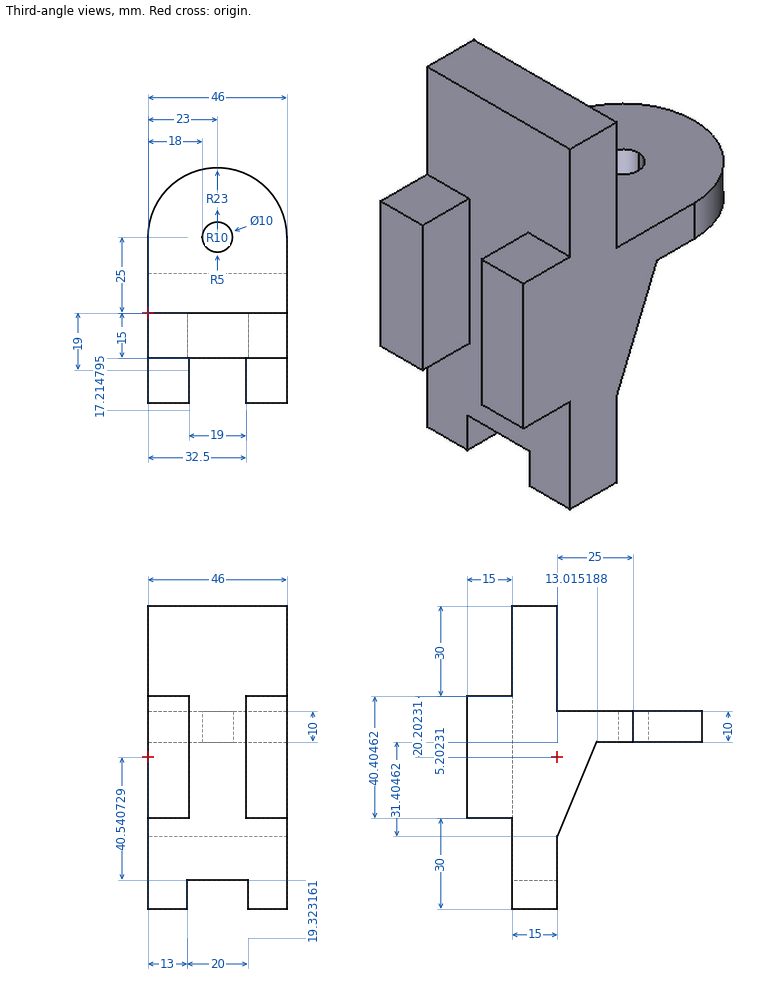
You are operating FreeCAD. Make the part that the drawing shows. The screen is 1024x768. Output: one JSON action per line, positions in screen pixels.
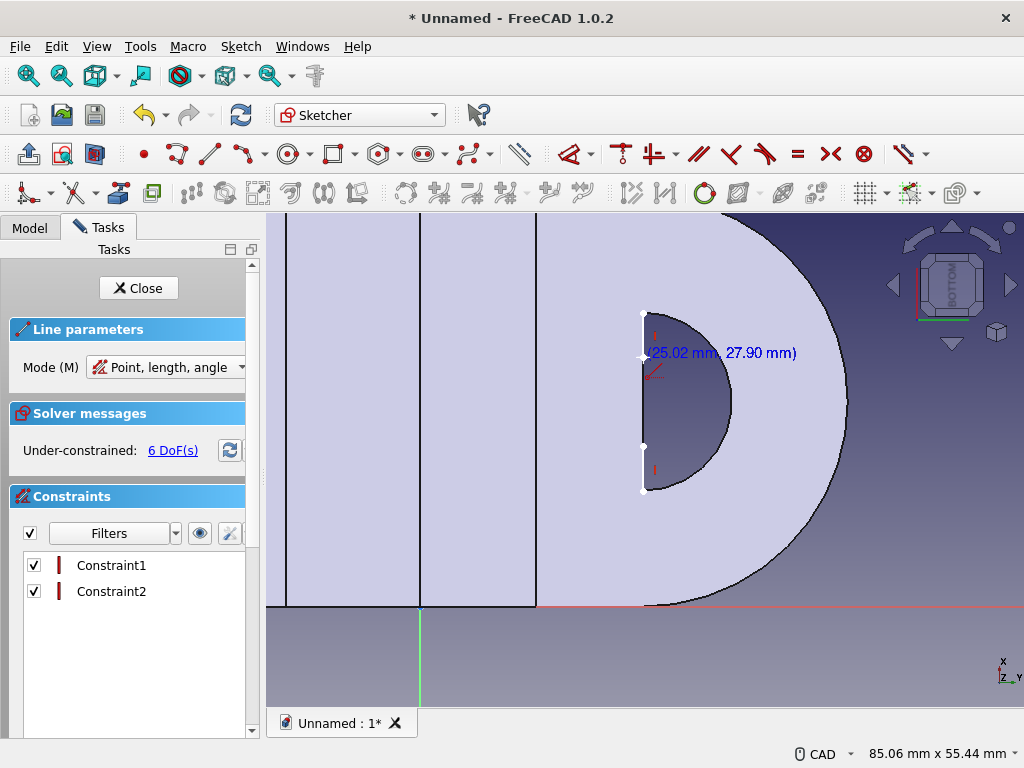
{"action": "key", "text": "g 3 a"}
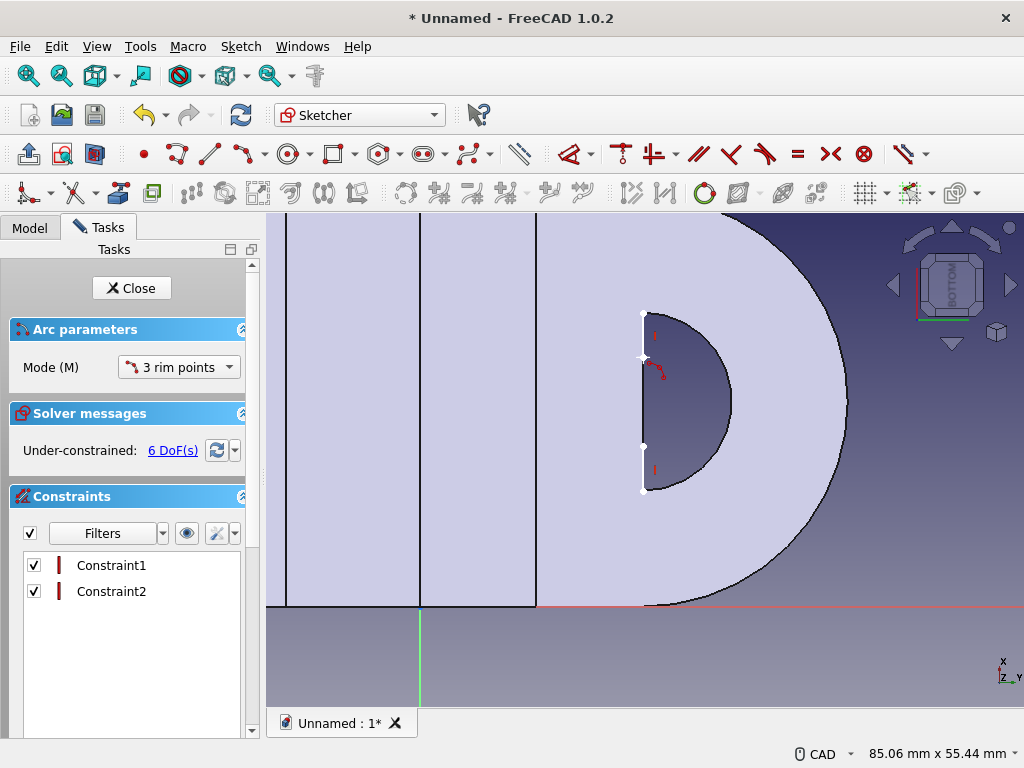
{"action": "left_click", "coordinate": [643, 492]}
{"action": "left_click", "coordinate": [643, 314]}
{"action": "left_click", "coordinate": [732, 402]}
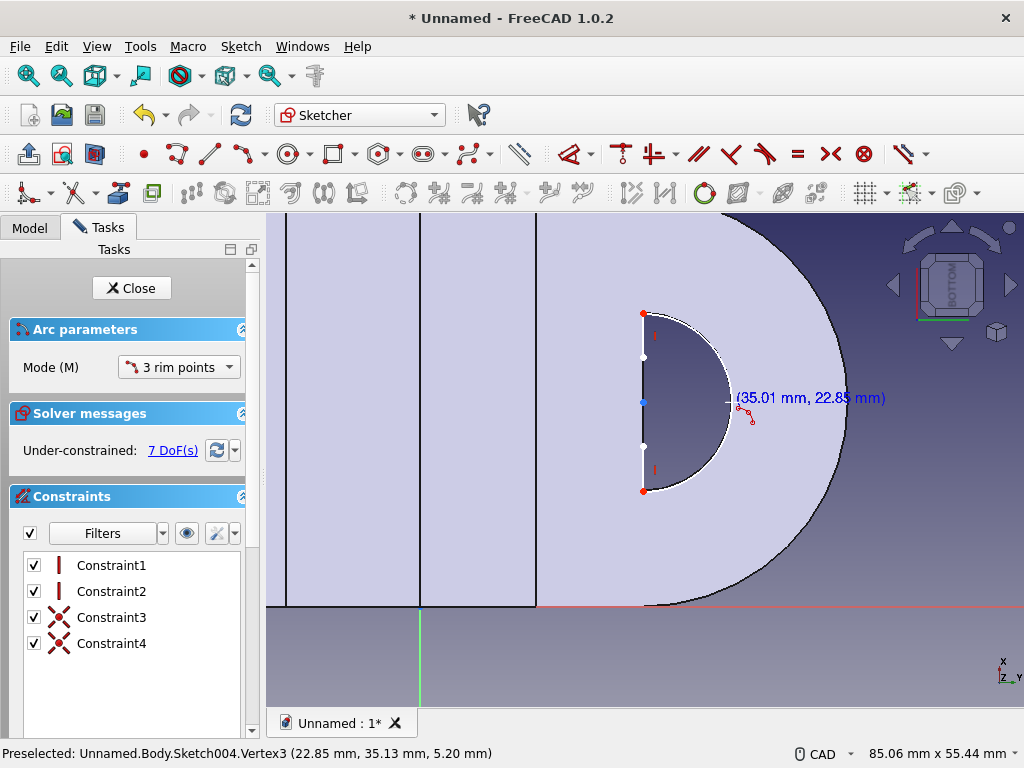
{"action": "left_click", "coordinate": [643, 358]}
{"action": "left_click", "coordinate": [643, 447]}
{"action": "left_click", "coordinate": [598, 402]}
{"action": "key", "text": "Escape"}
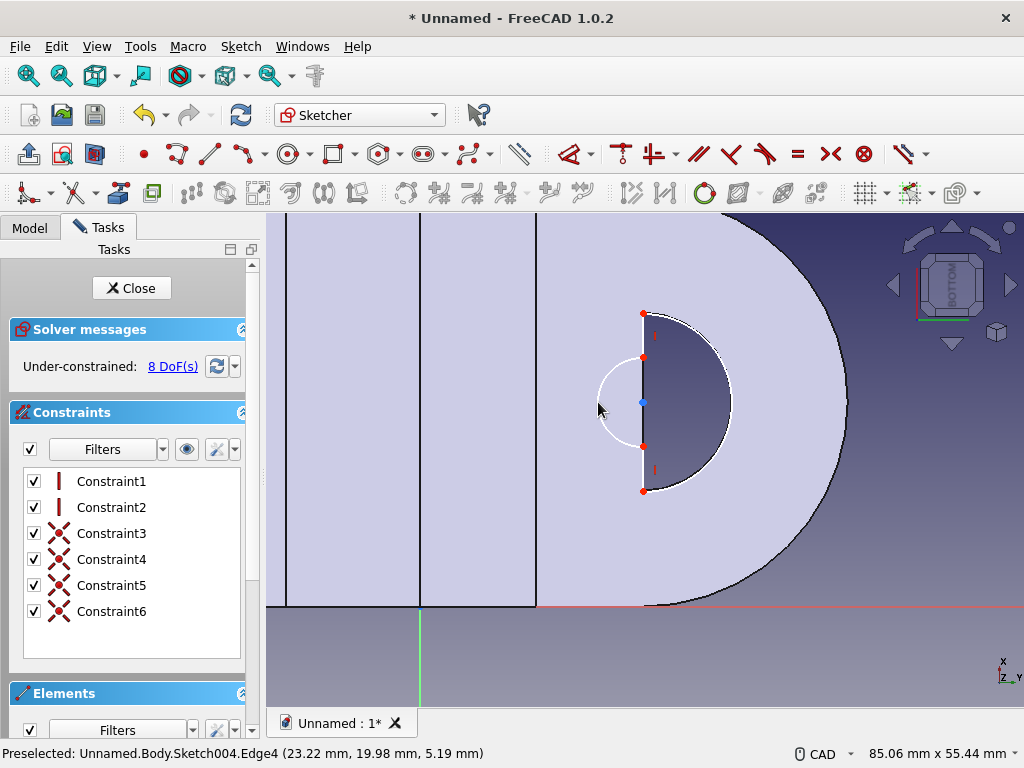
{"action": "left_click", "coordinate": [715, 455]}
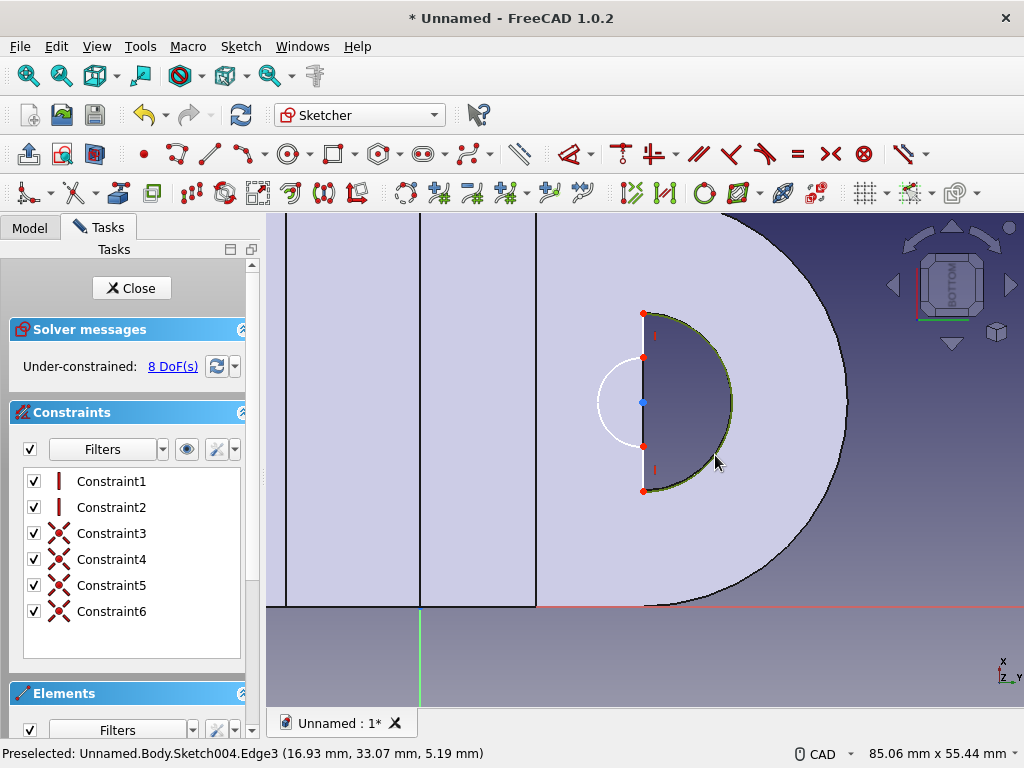
{"action": "left_click", "coordinate": [607, 376]}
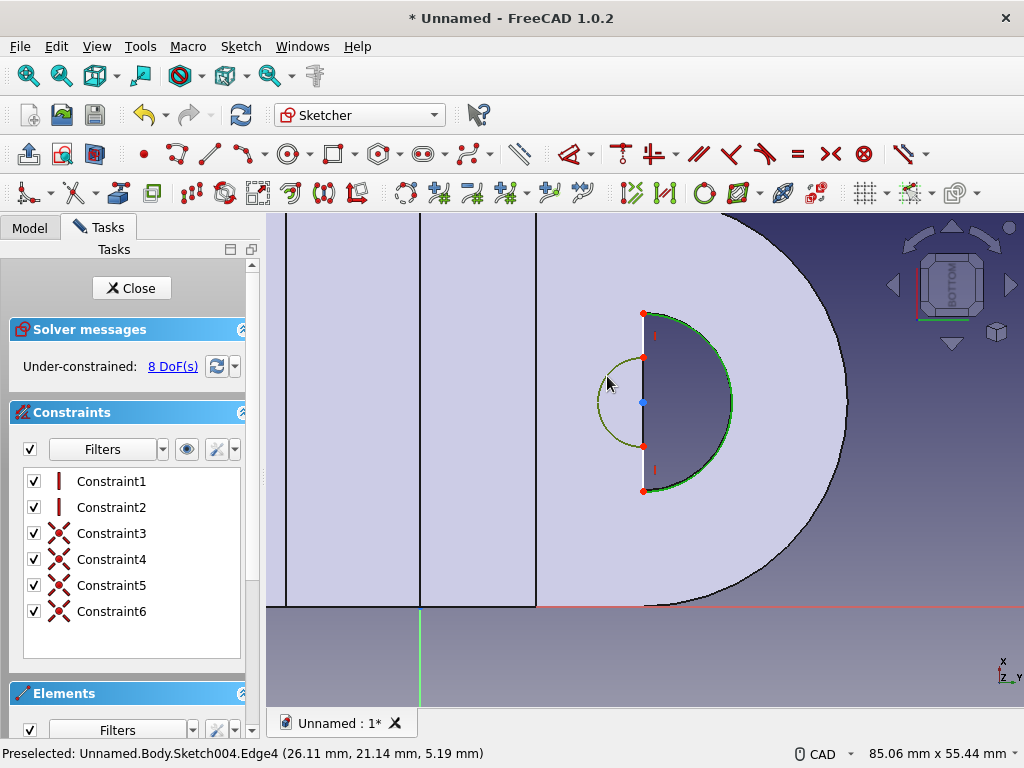
{"action": "key", "text": "c"}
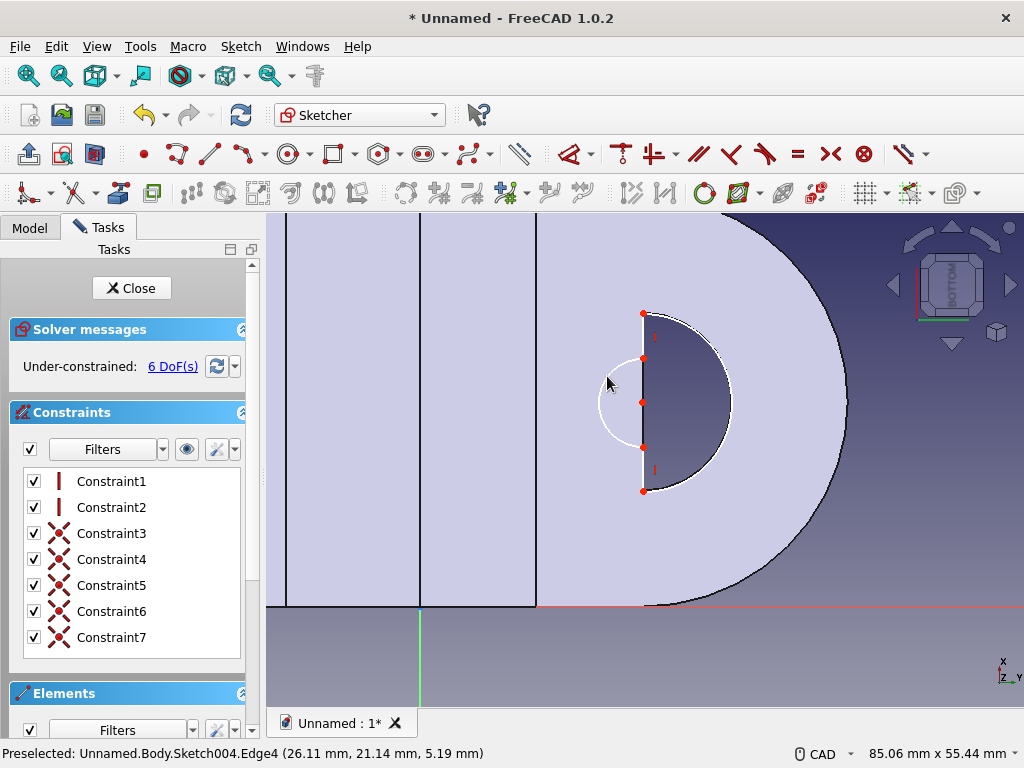
{"action": "key", "text": "d"}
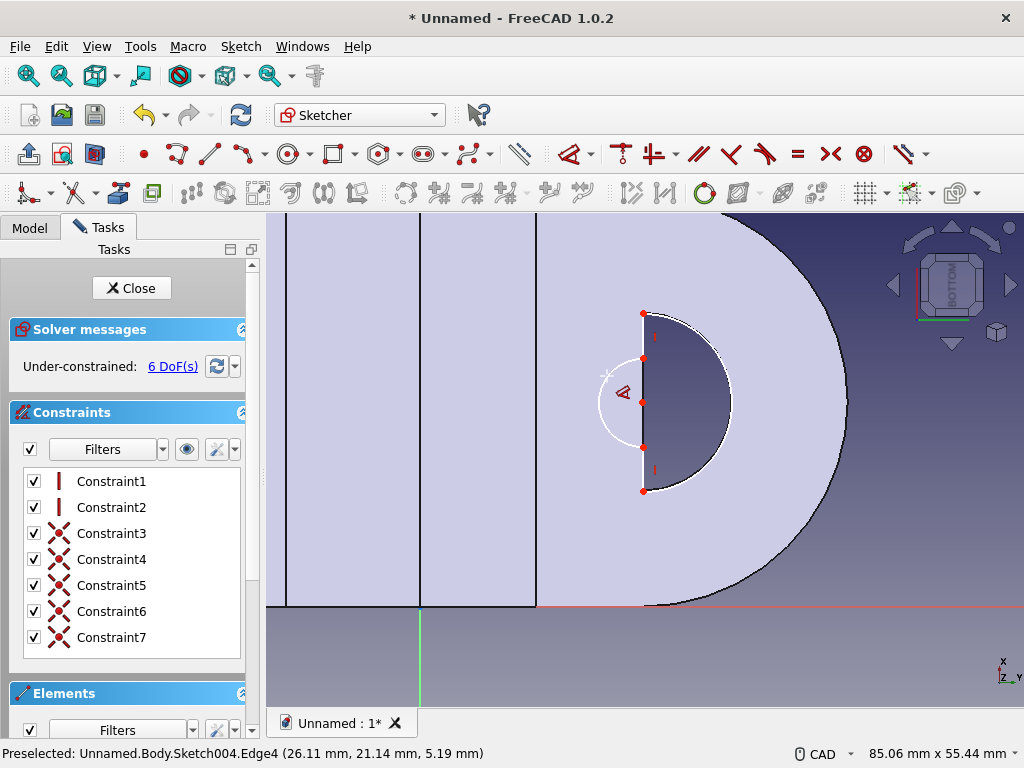
{"action": "left_click", "coordinate": [715, 455]}
{"action": "left_click", "coordinate": [741, 474]}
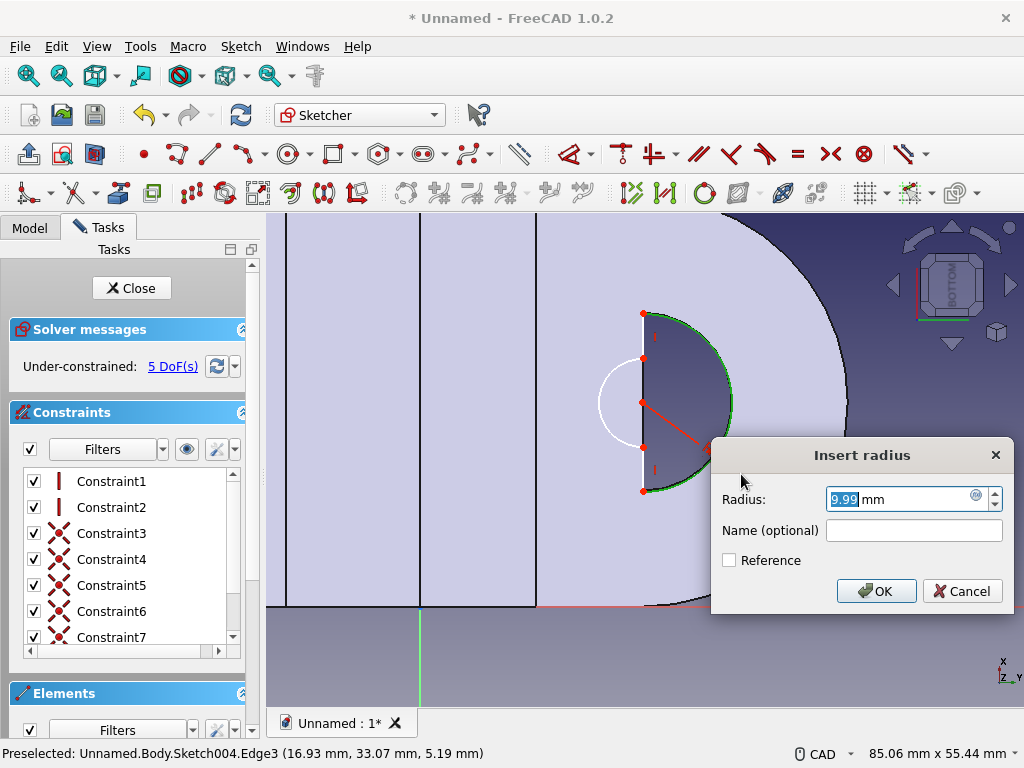
{"action": "type", "text": "10"}
{"action": "key", "text": "Return"}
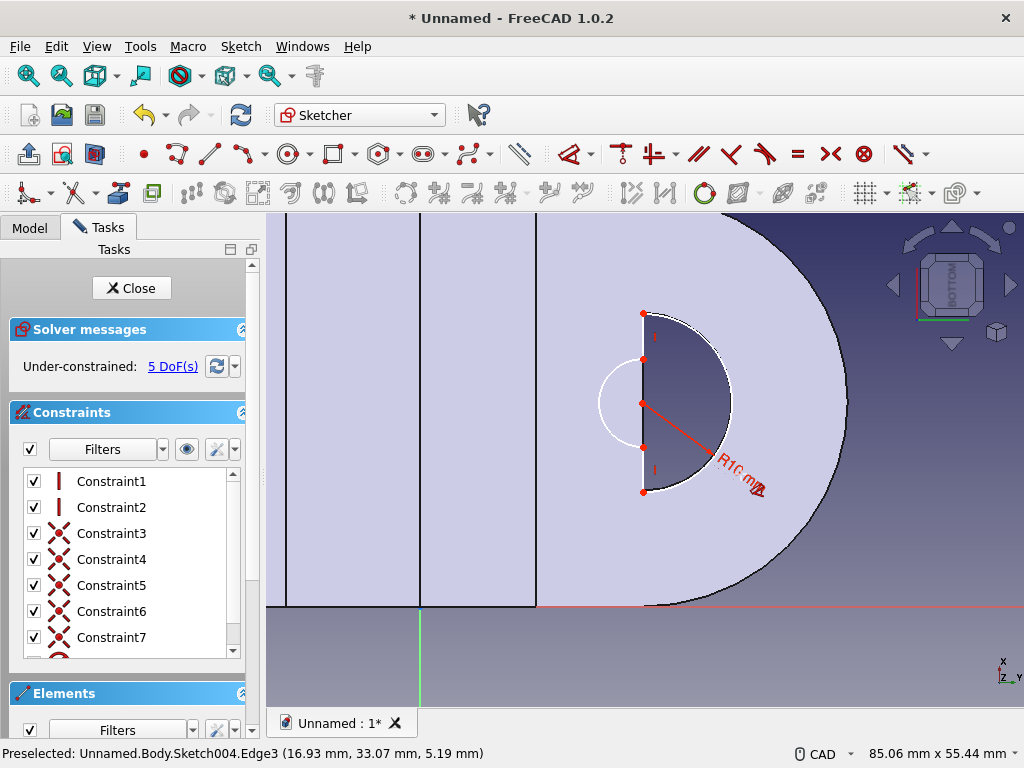
{"action": "left_click", "coordinate": [607, 377]}
{"action": "left_click", "coordinate": [581, 358]}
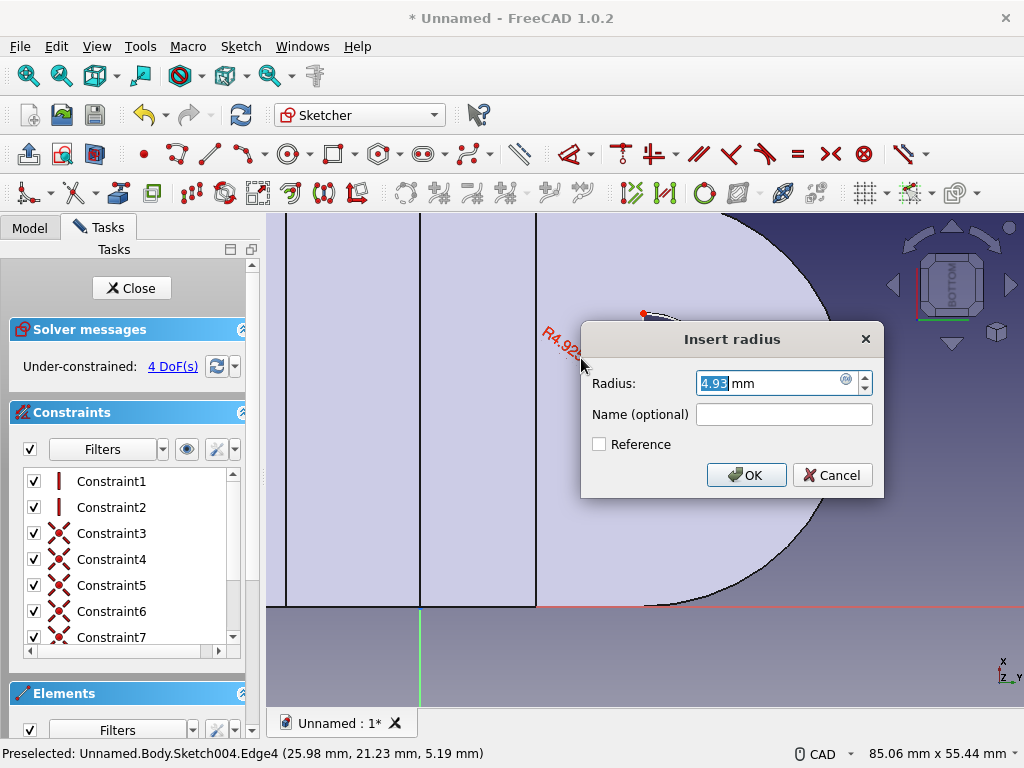
{"action": "type", "text": "5"}
{"action": "key", "text": "Return"}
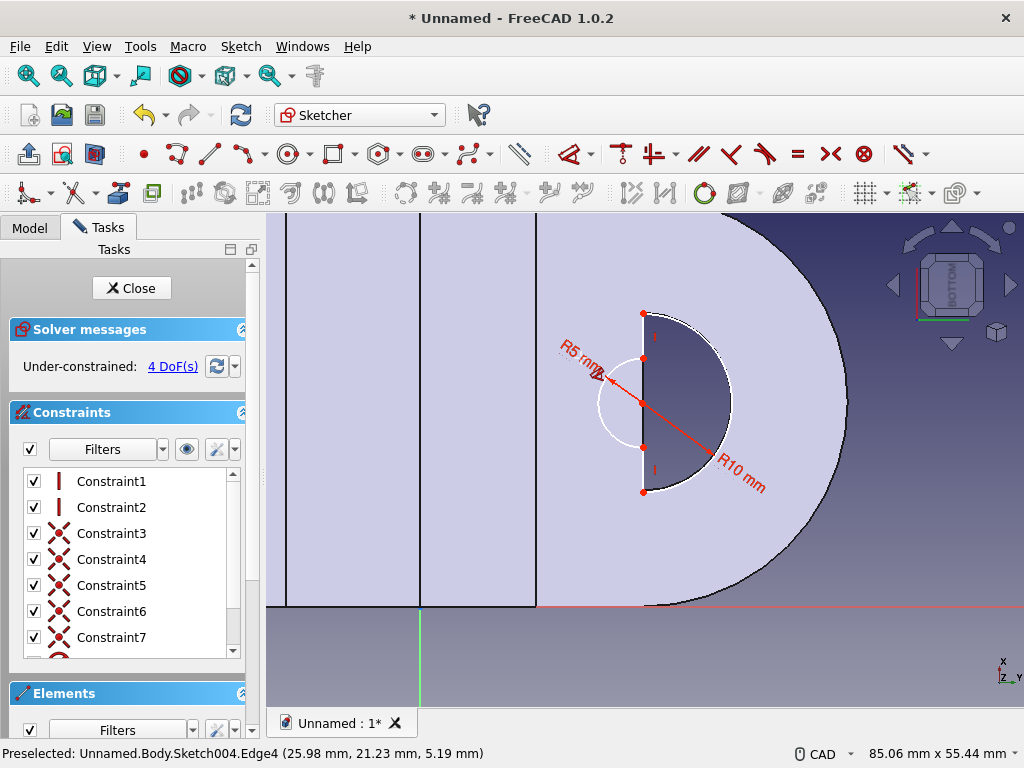
{"action": "left_click", "coordinate": [643, 448]}
{"action": "left_click", "coordinate": [532, 641]}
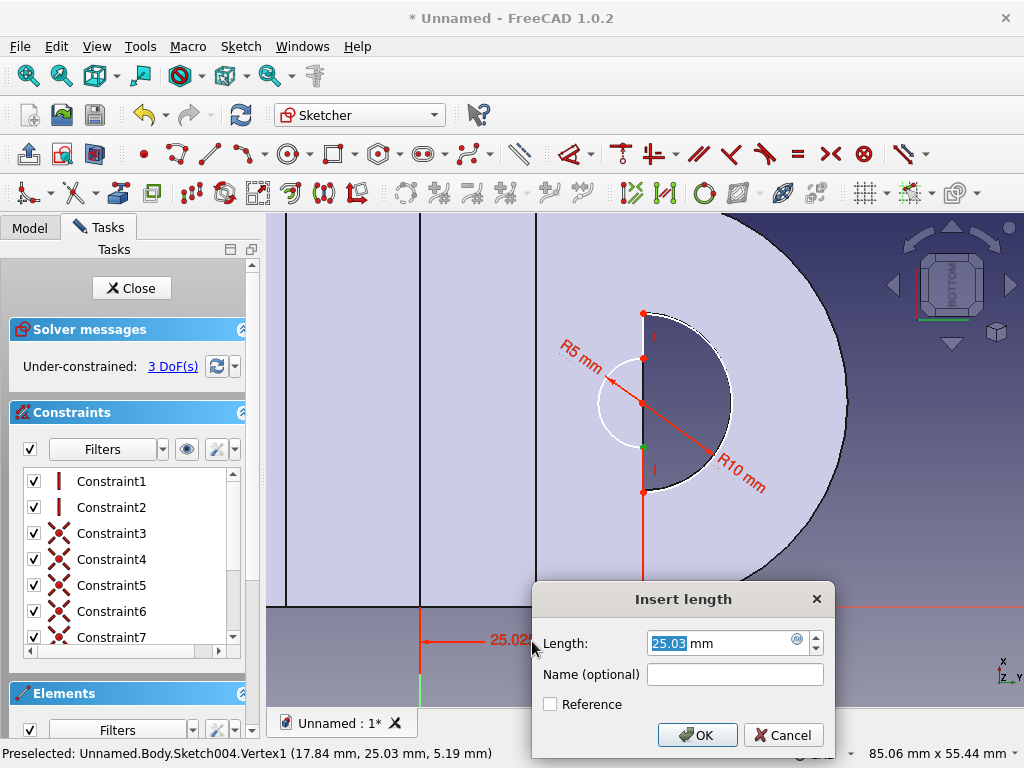
{"action": "type", "text": "25"}
{"action": "key", "text": "Return"}